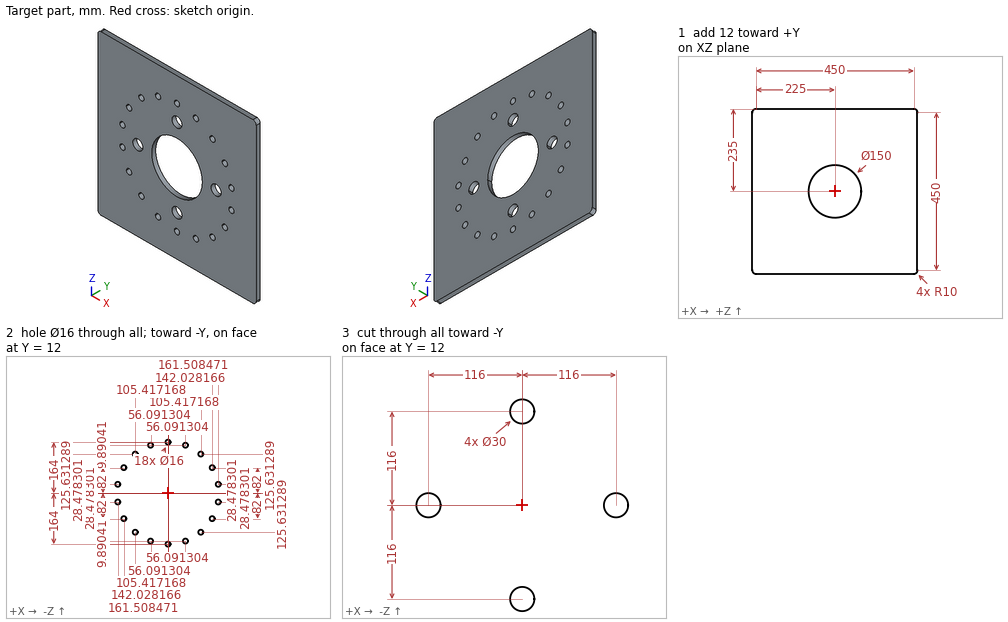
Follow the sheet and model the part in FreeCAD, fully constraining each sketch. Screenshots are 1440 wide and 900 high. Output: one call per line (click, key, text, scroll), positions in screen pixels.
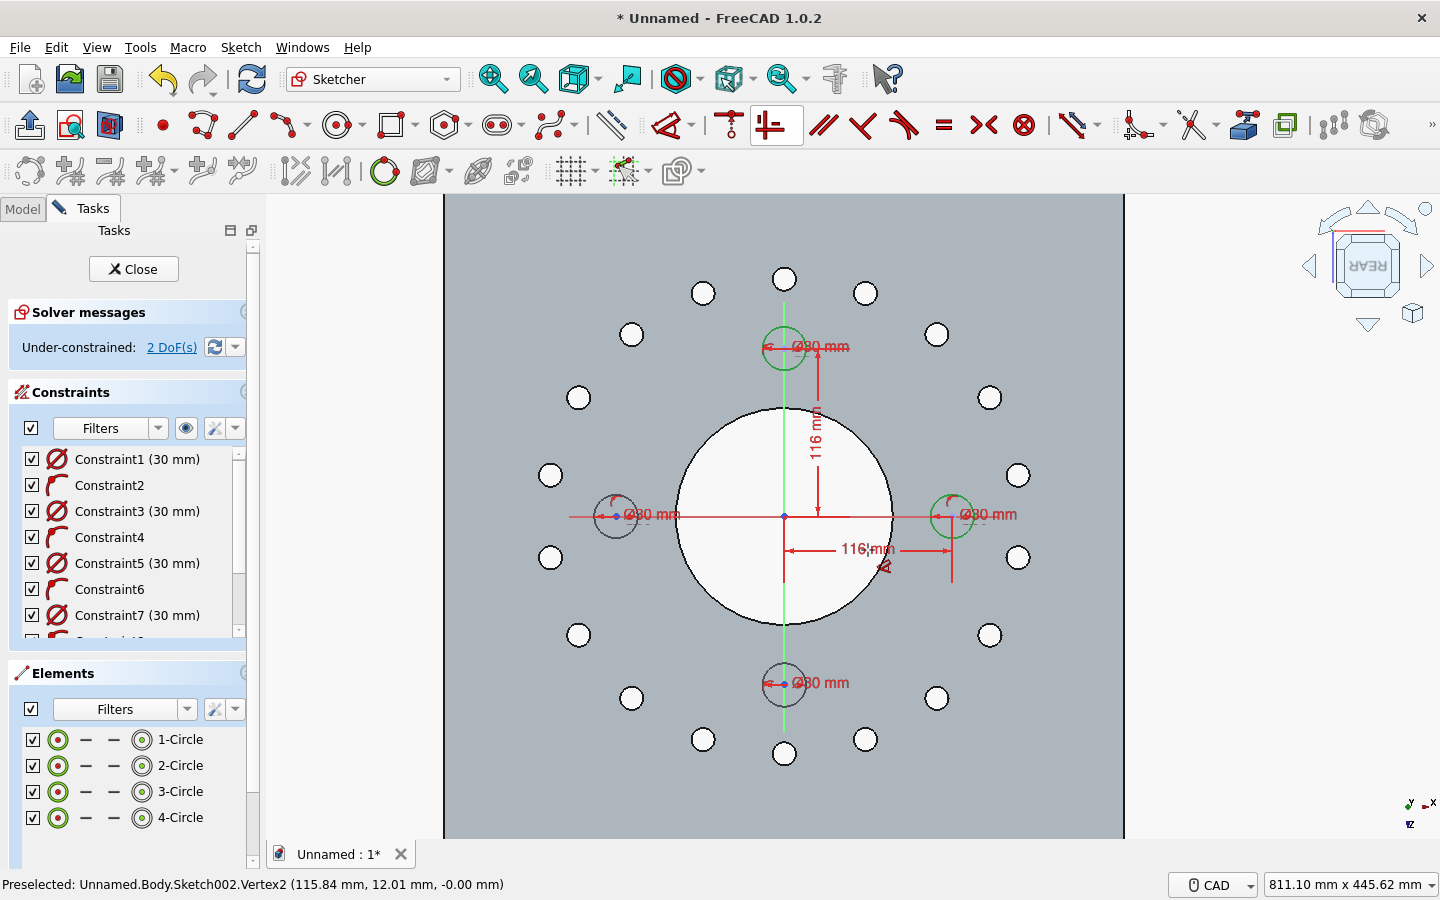
click(784, 685)
click(818, 601)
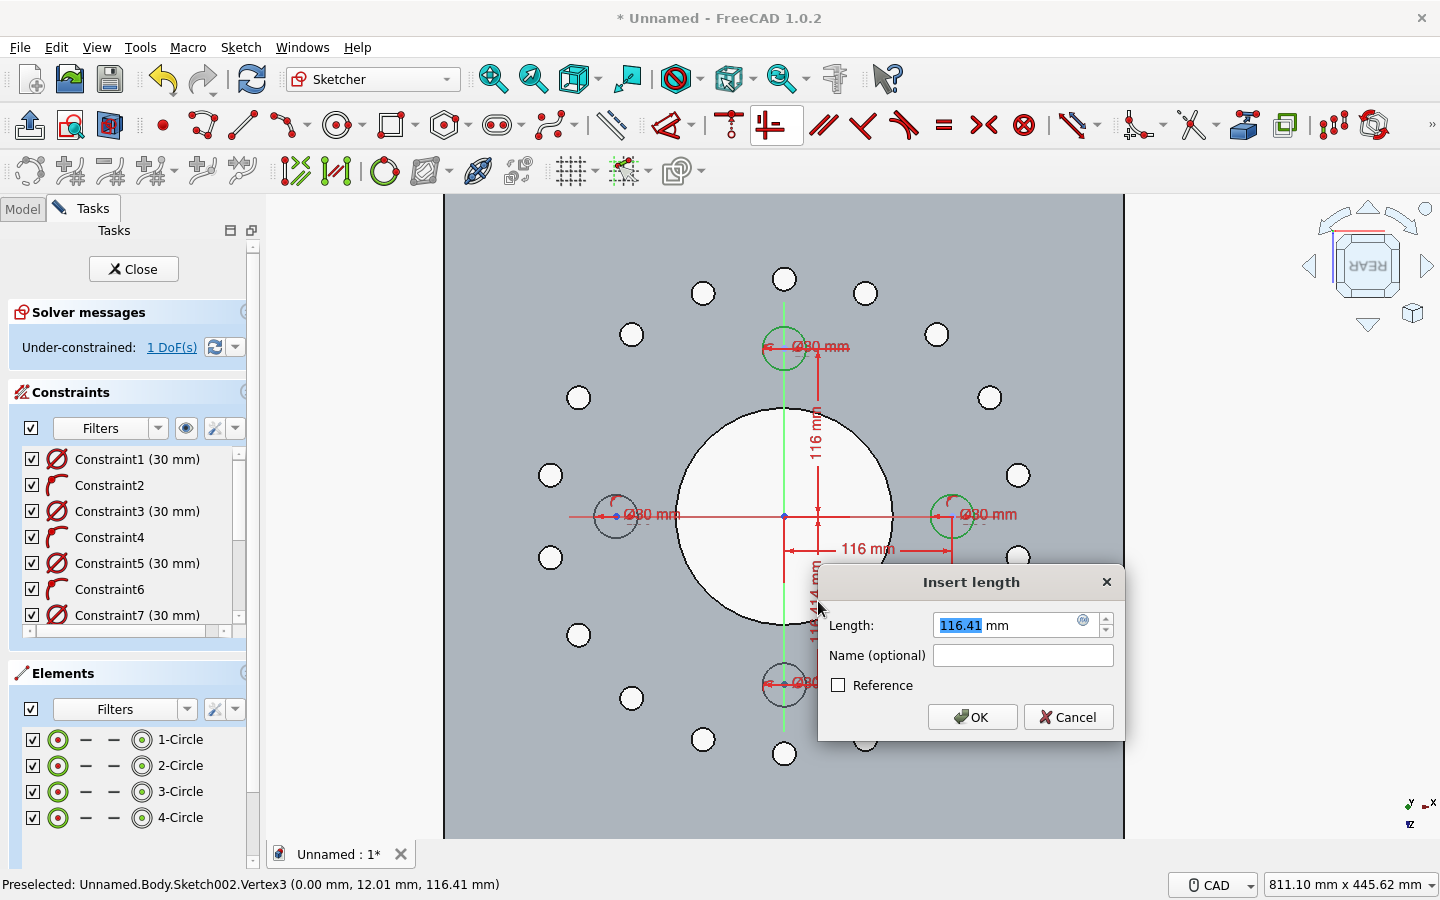
text(116)
key(Return)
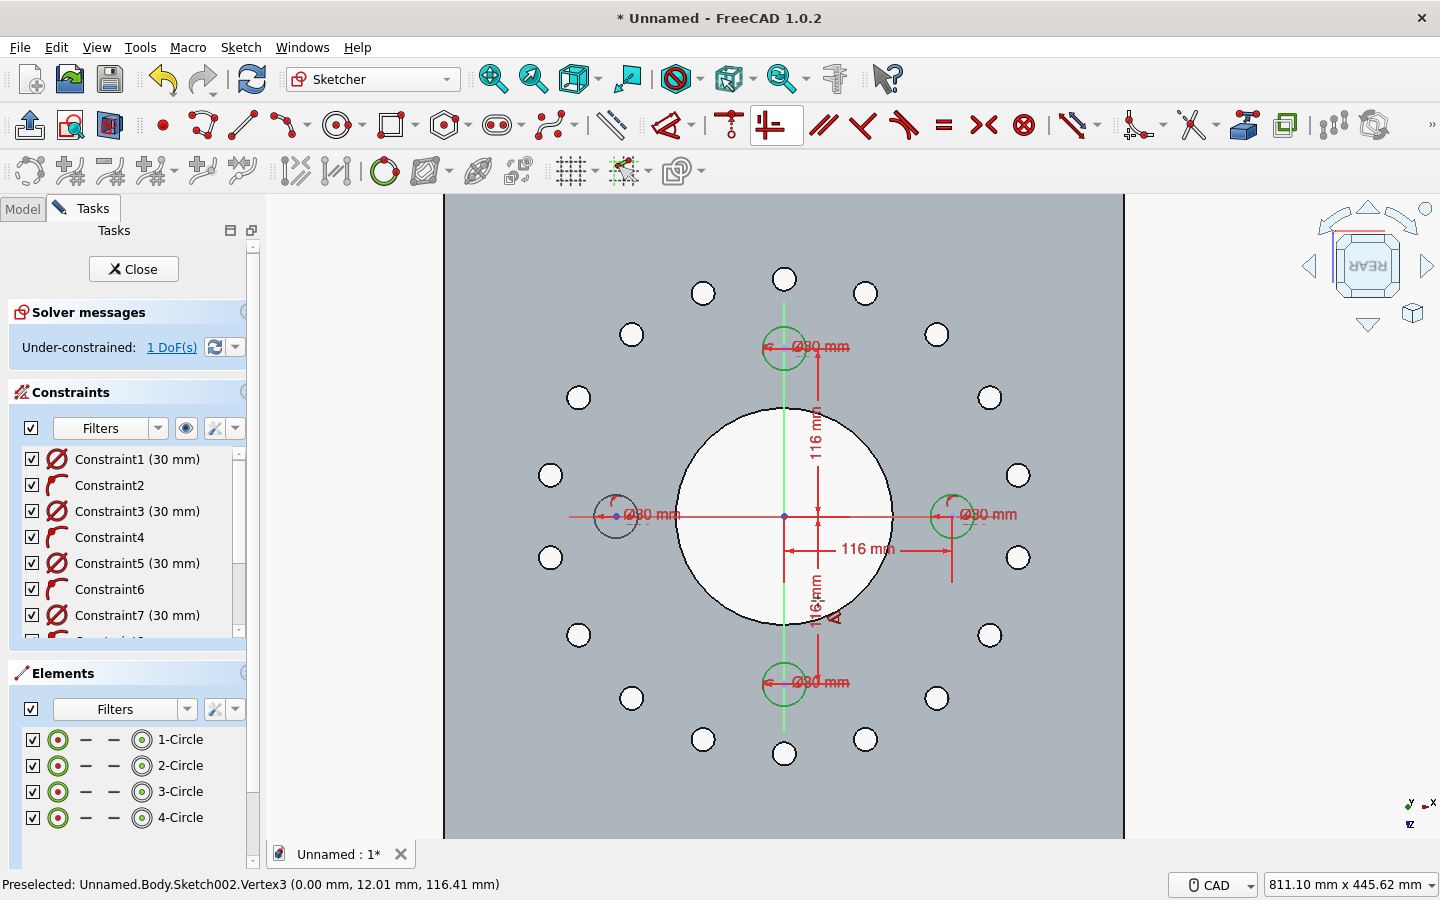
click(616, 516)
click(700, 550)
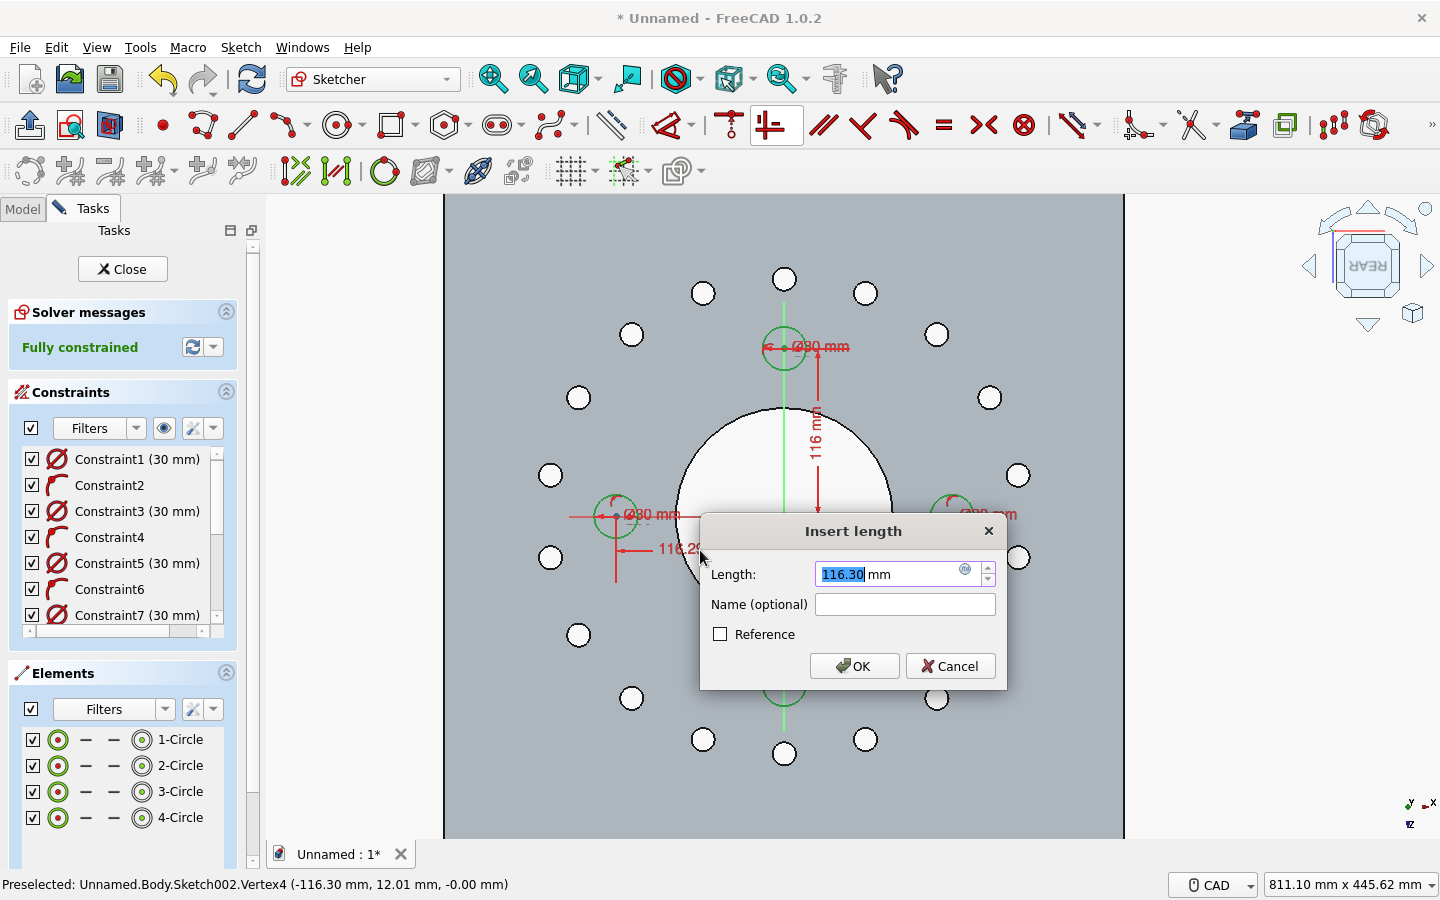
text(116)
key(Return)
key(Escape)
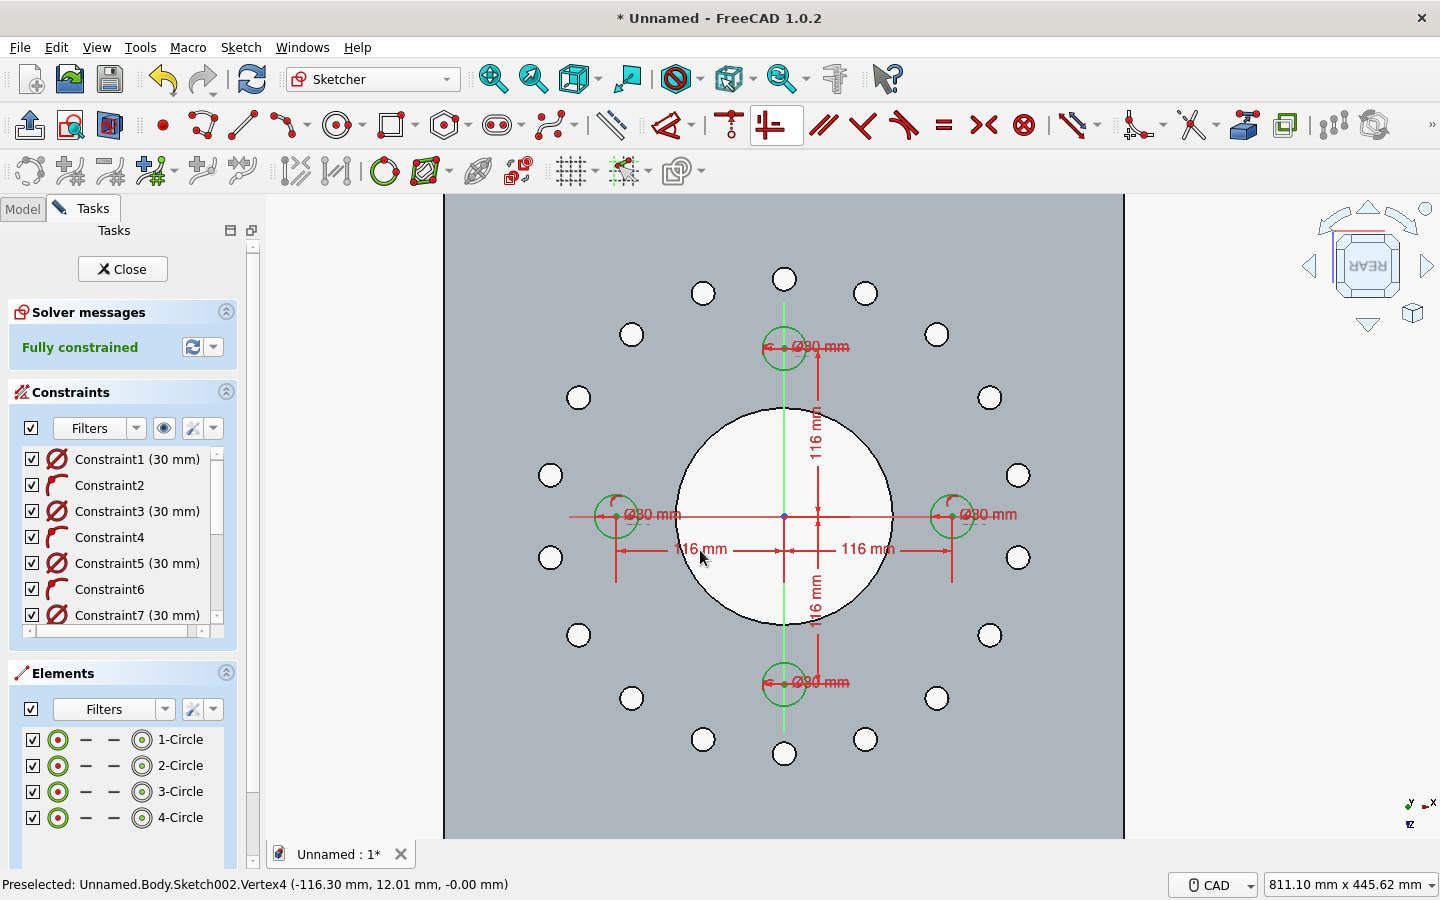
click(123, 269)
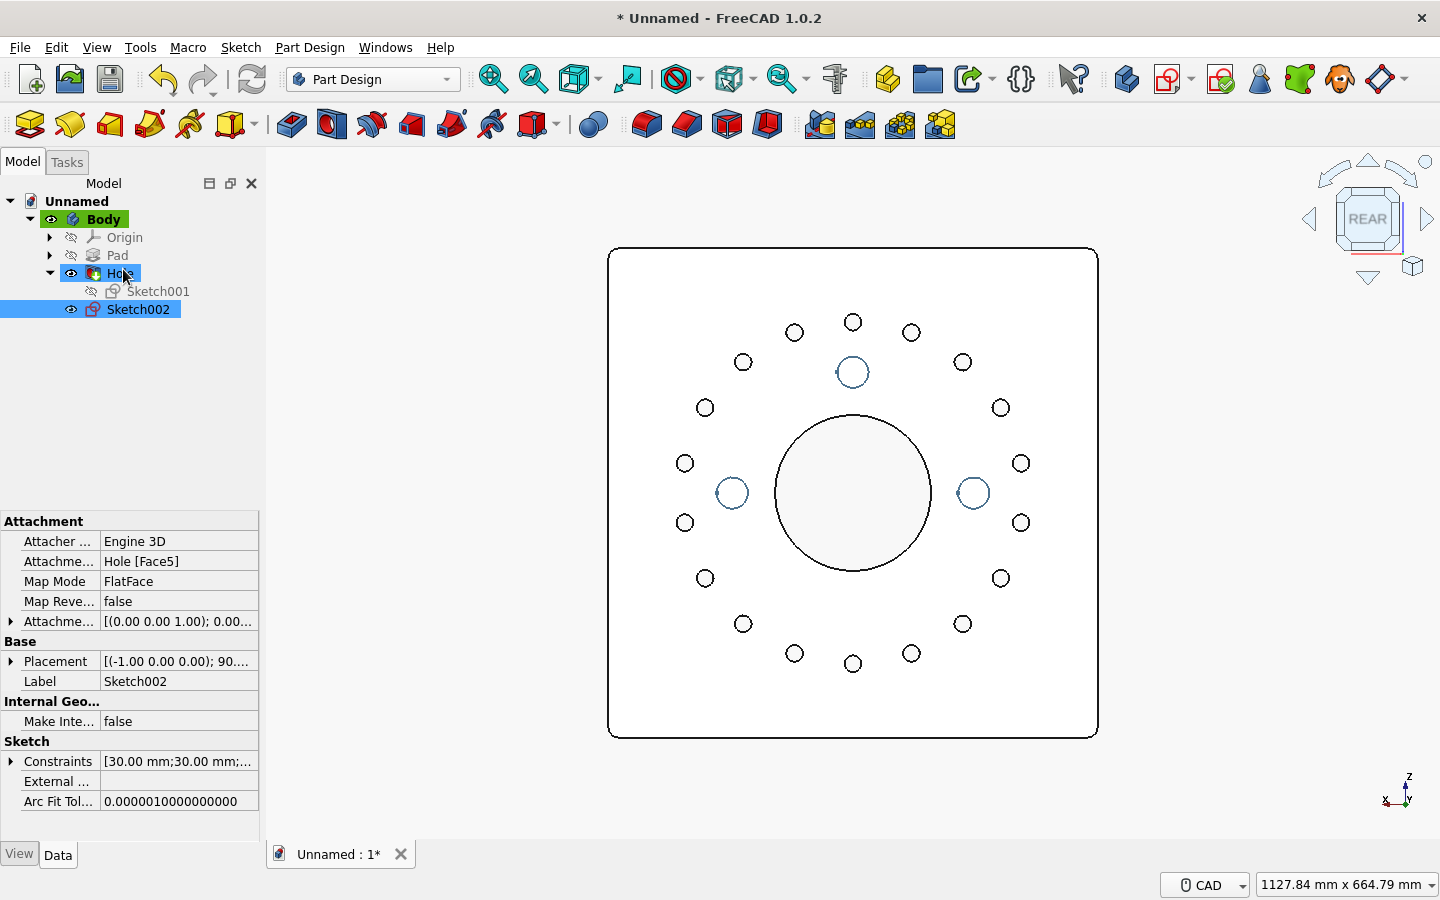
click(292, 124)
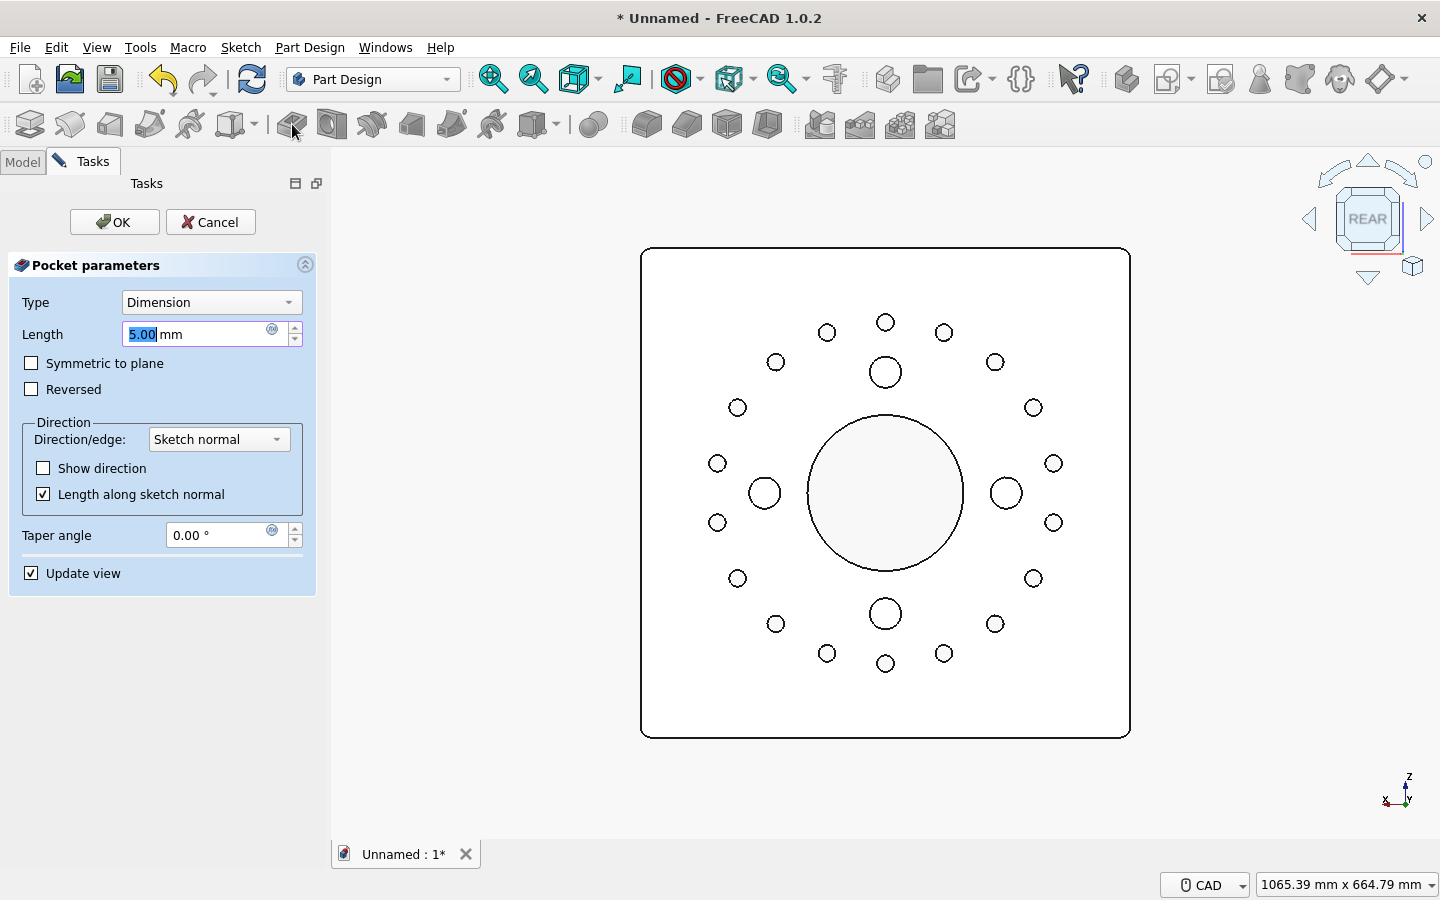
click(212, 302)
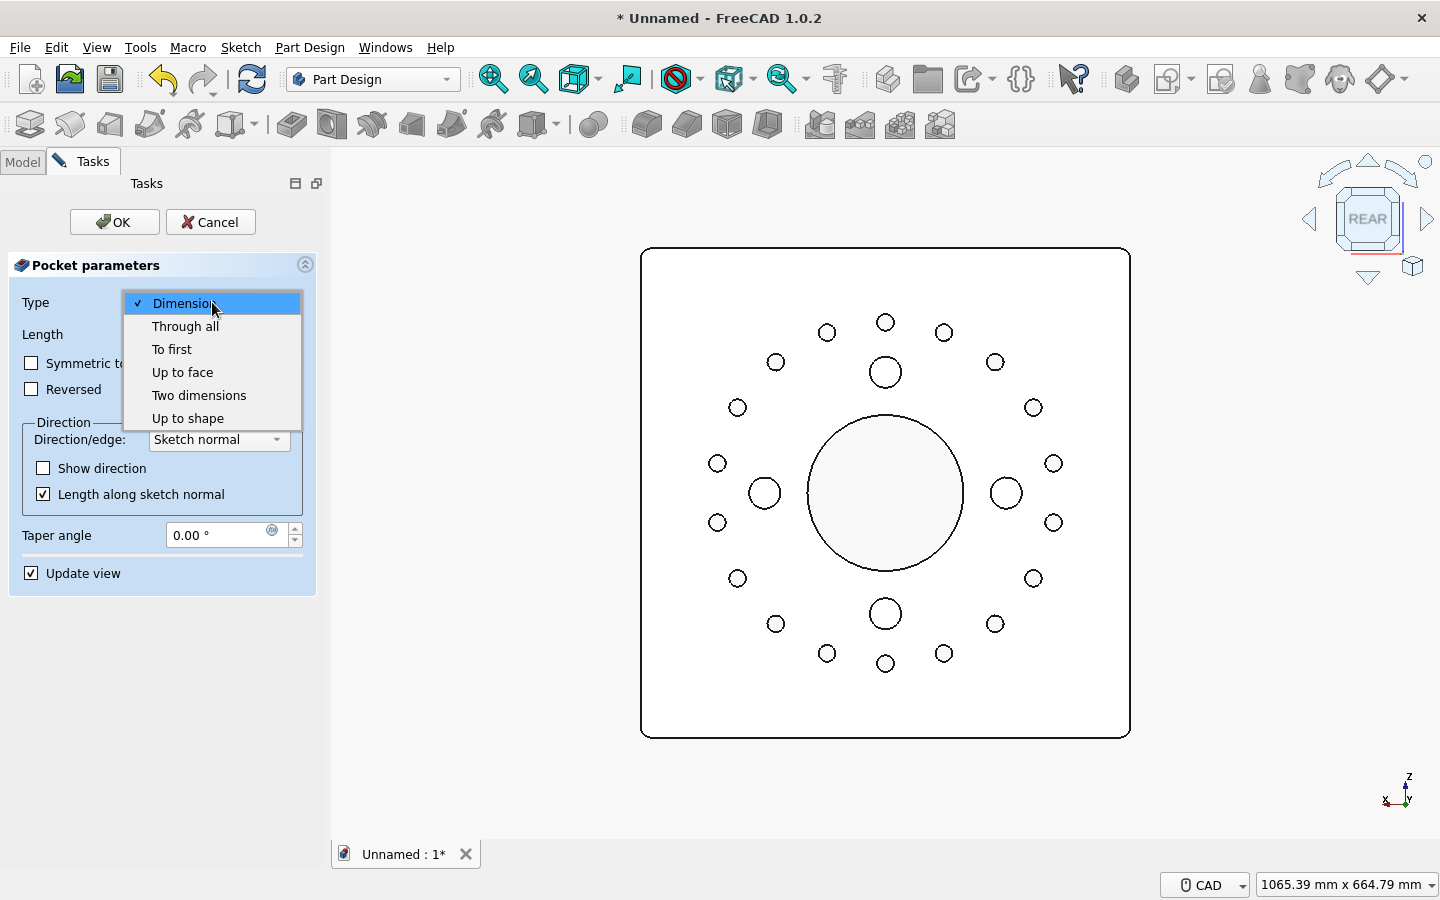
click(212, 326)